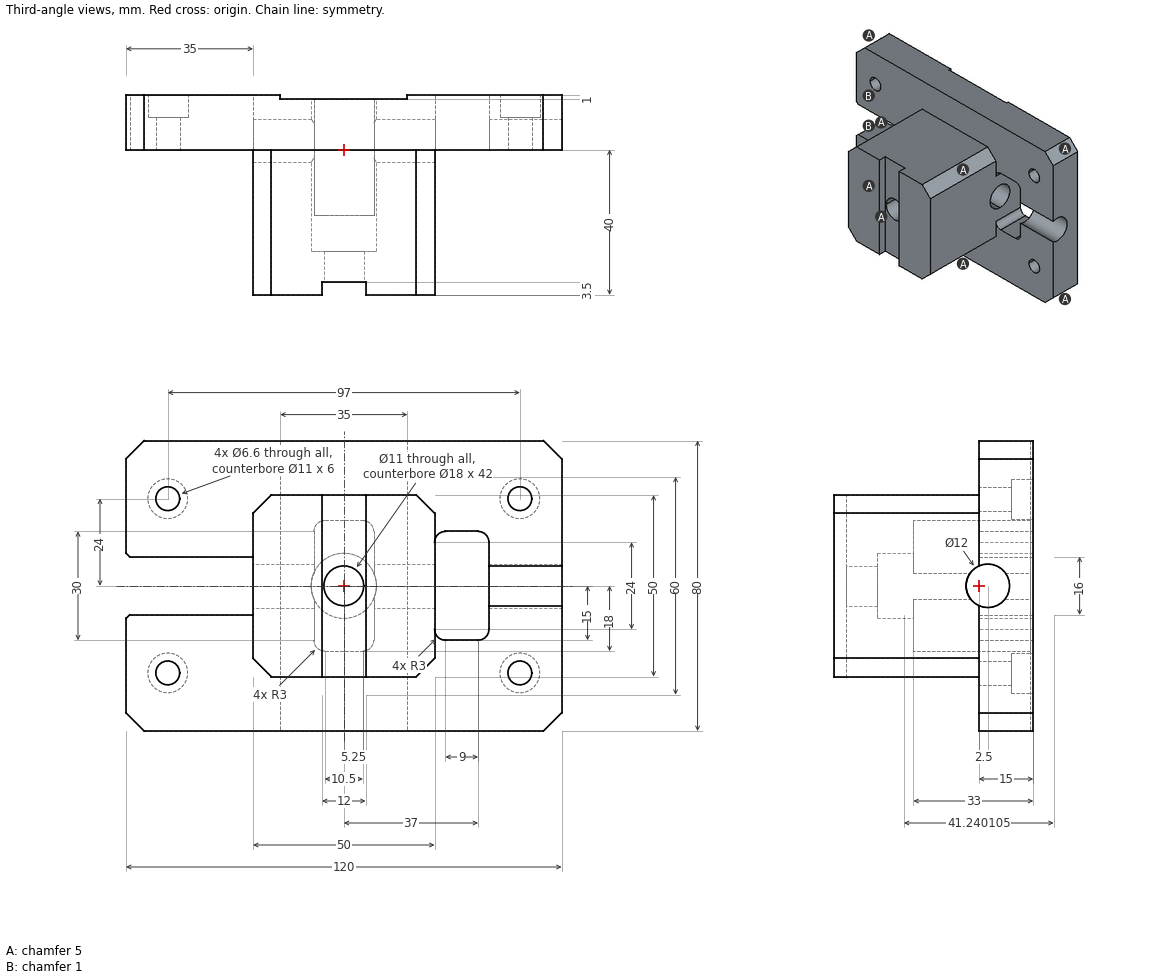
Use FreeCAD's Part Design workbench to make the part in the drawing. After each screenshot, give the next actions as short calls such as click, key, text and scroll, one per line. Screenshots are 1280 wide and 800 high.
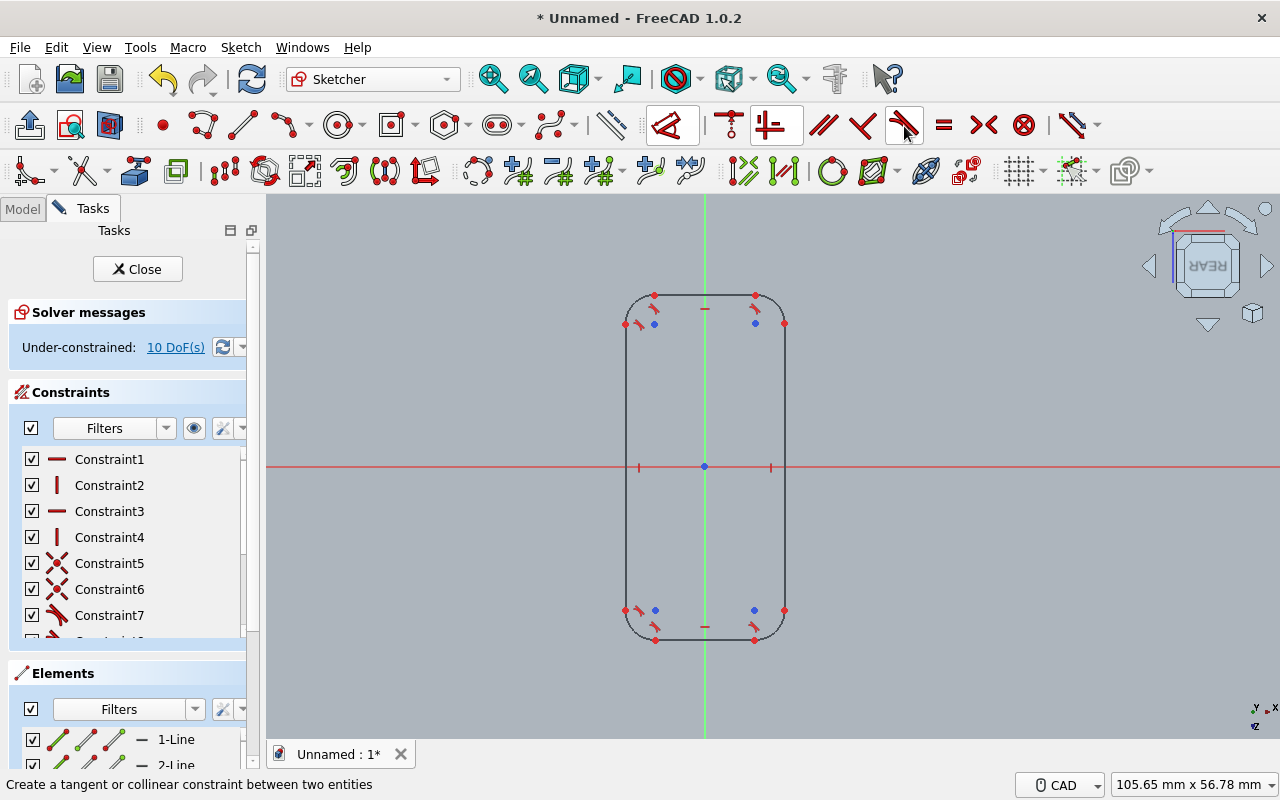
click(785, 525)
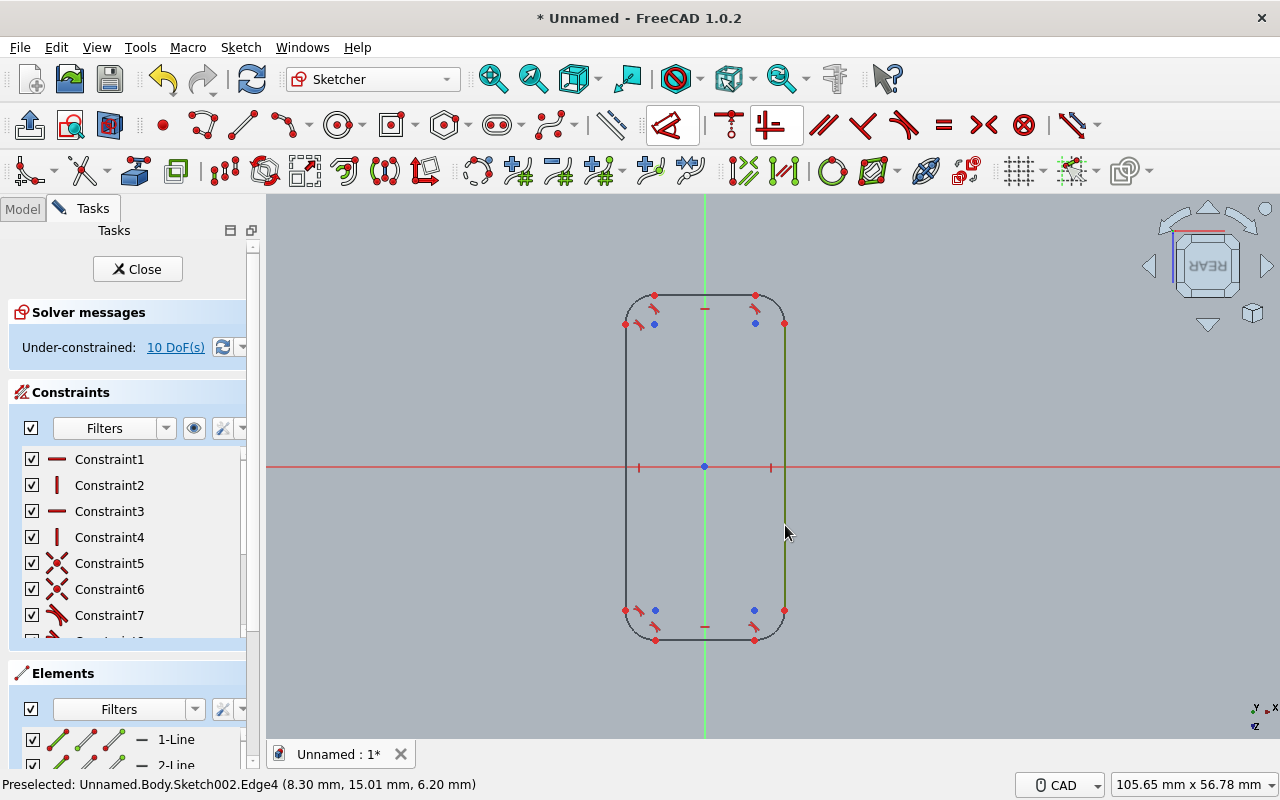
click(768, 637)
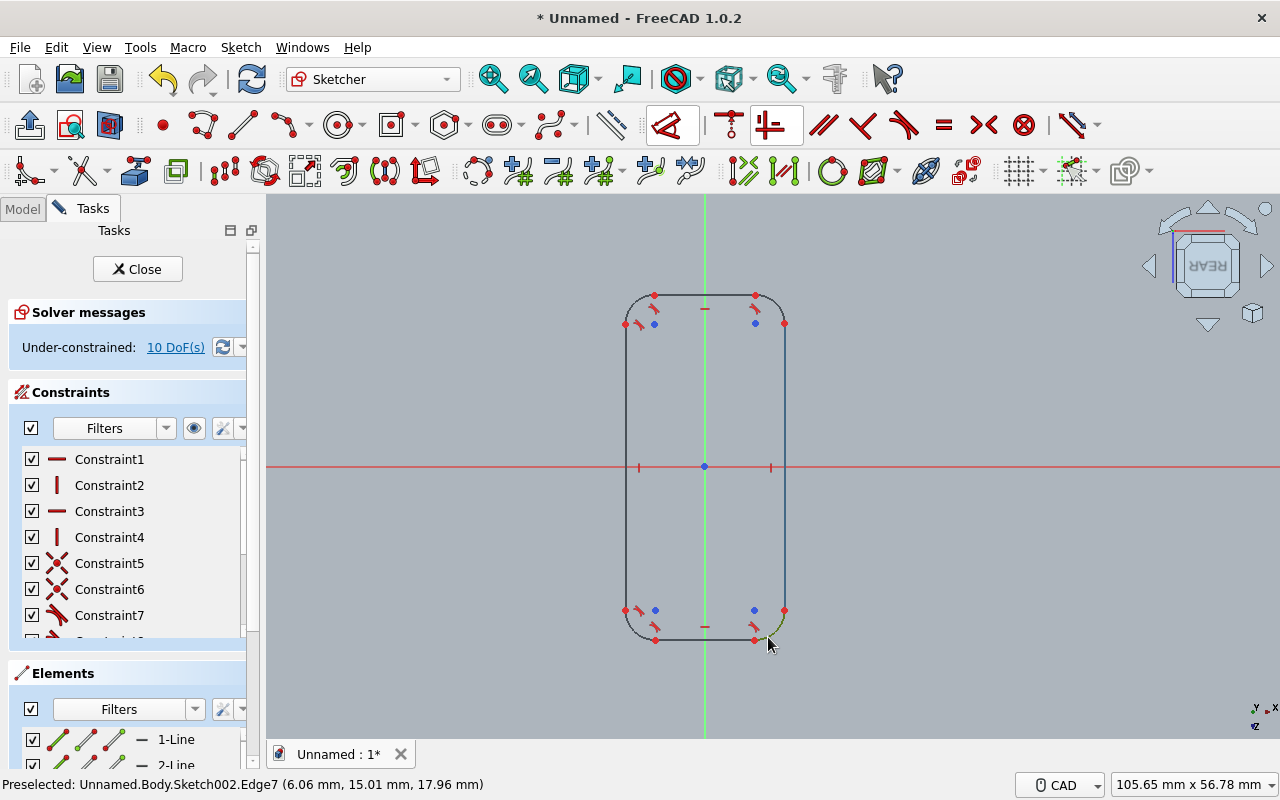
click(904, 126)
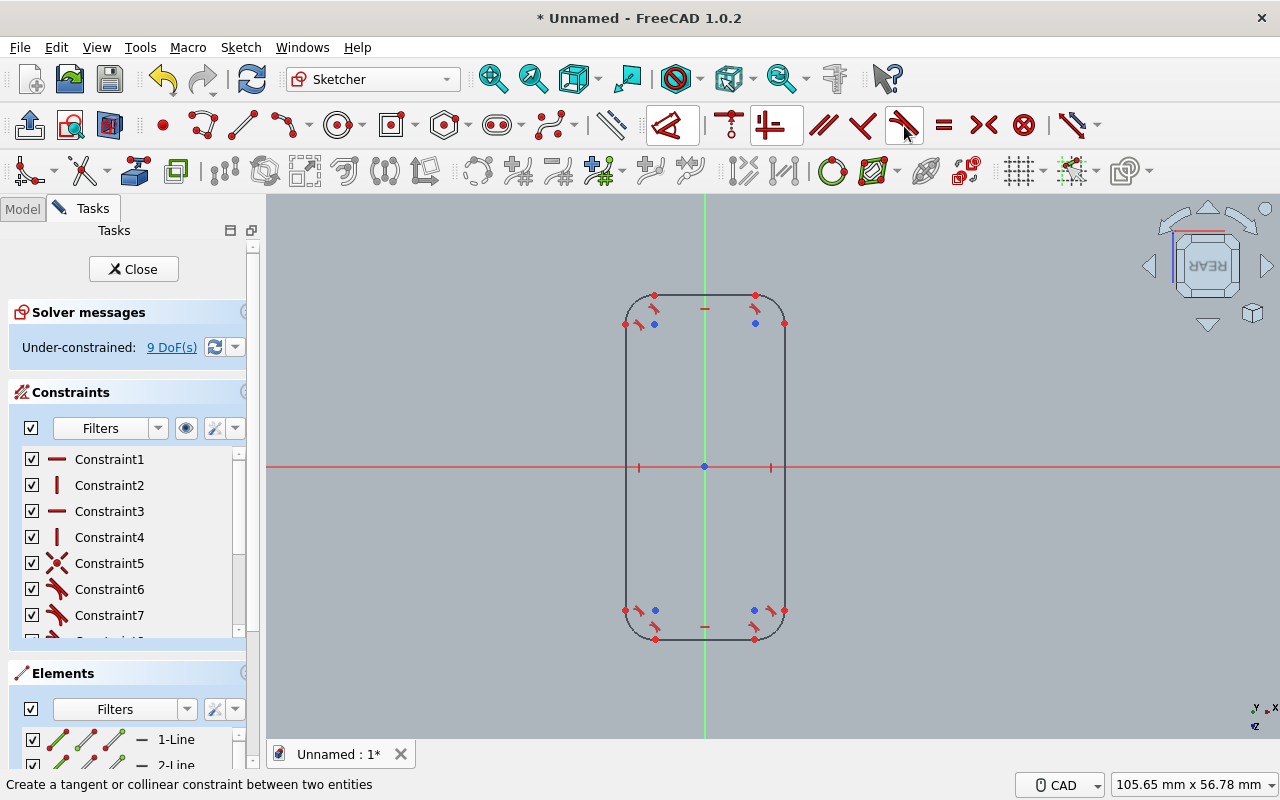
click(785, 524)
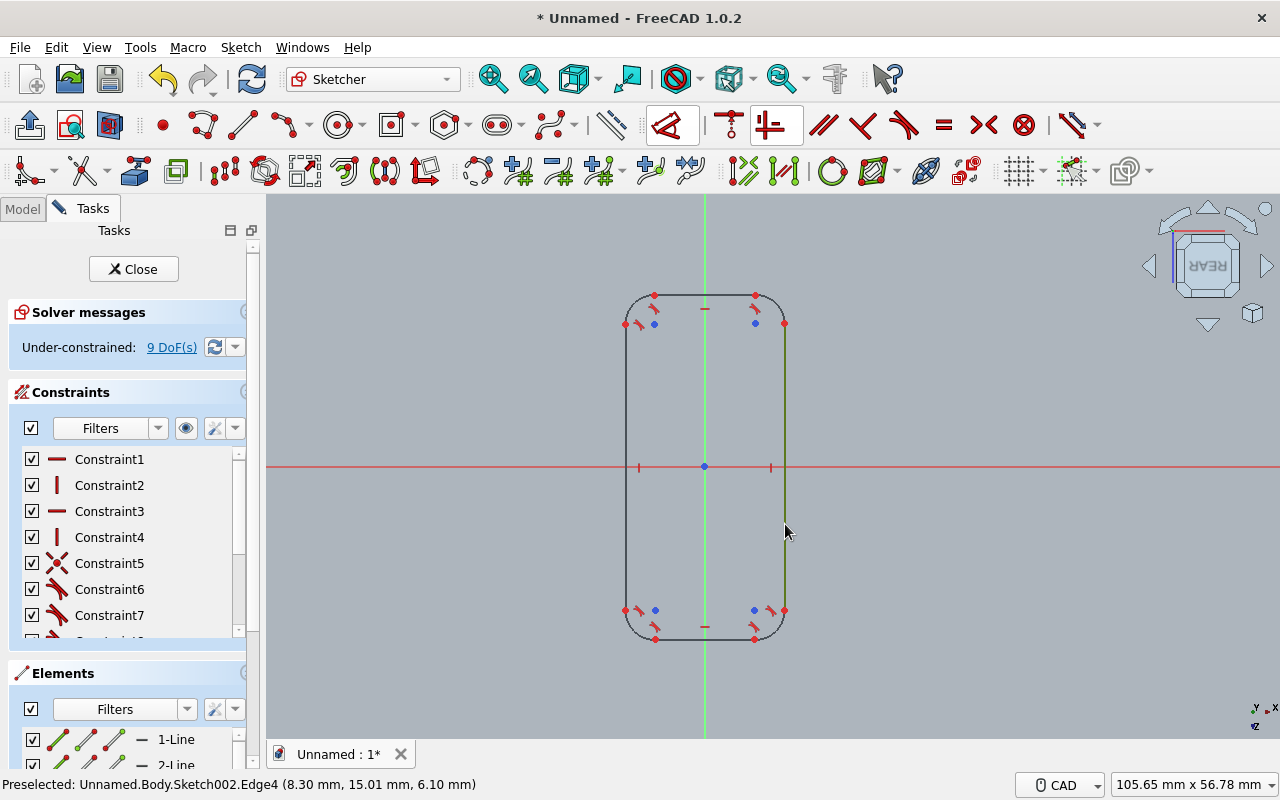
click(781, 311)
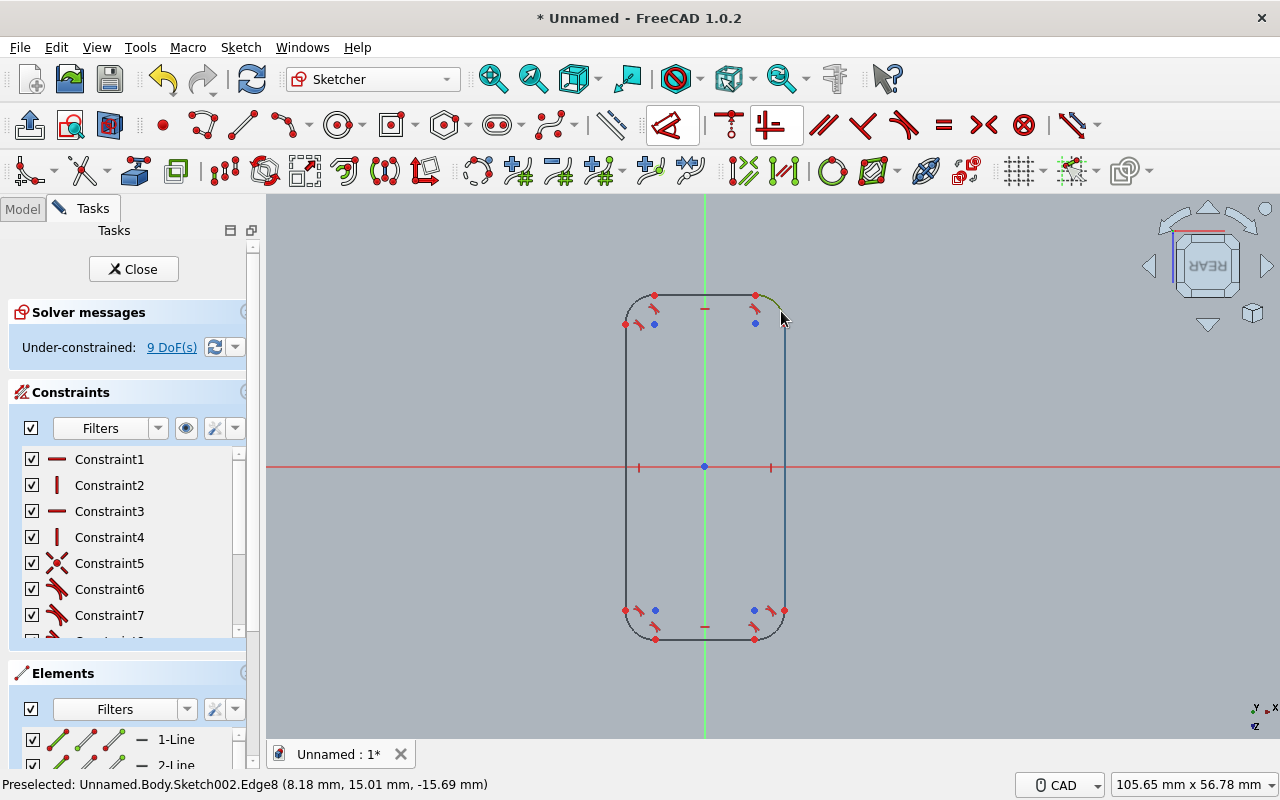
click(904, 126)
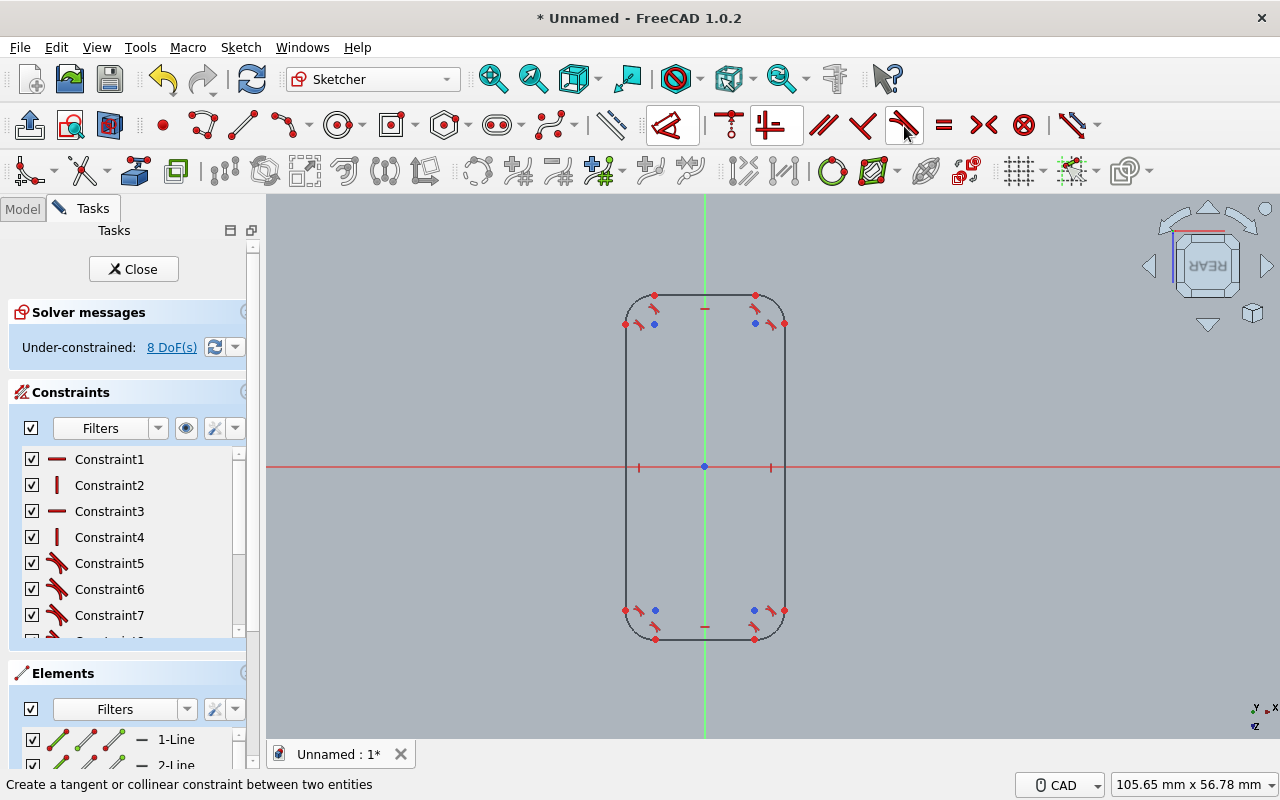
click(641, 298)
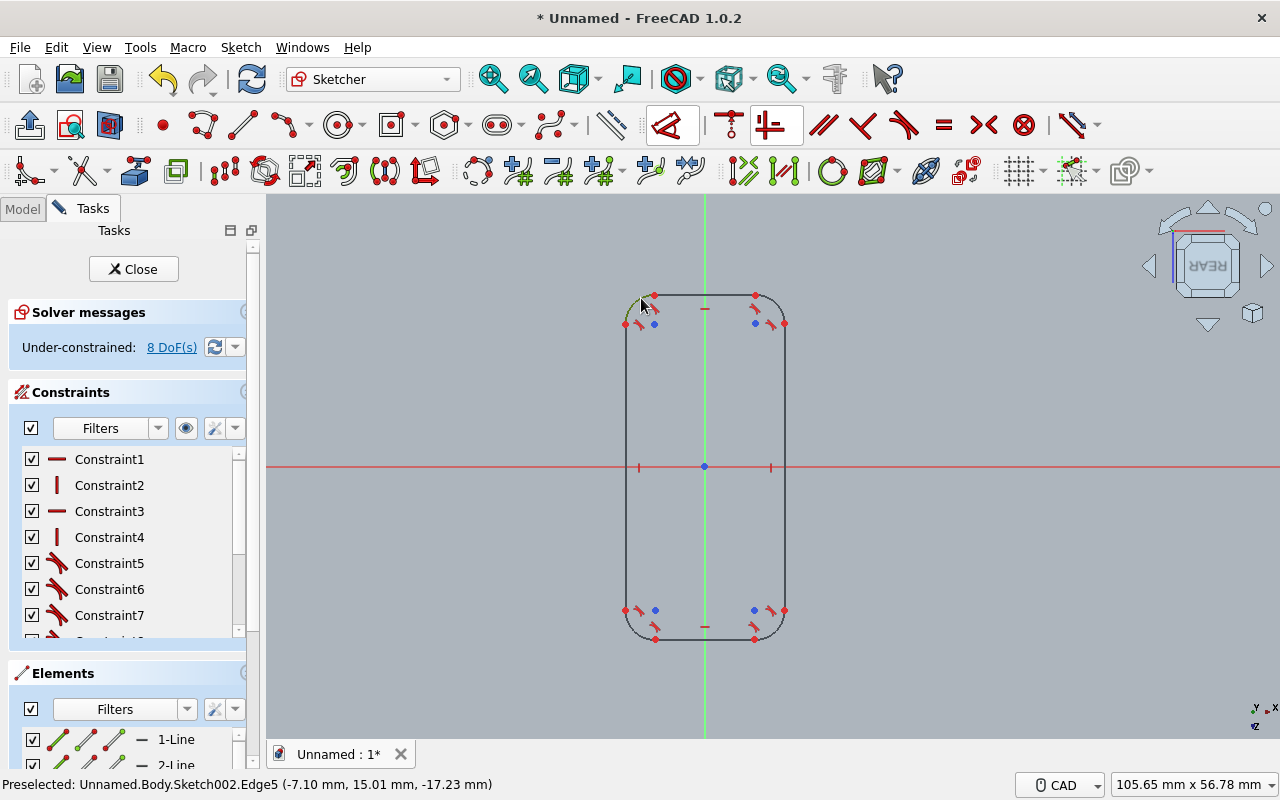
click(629, 624)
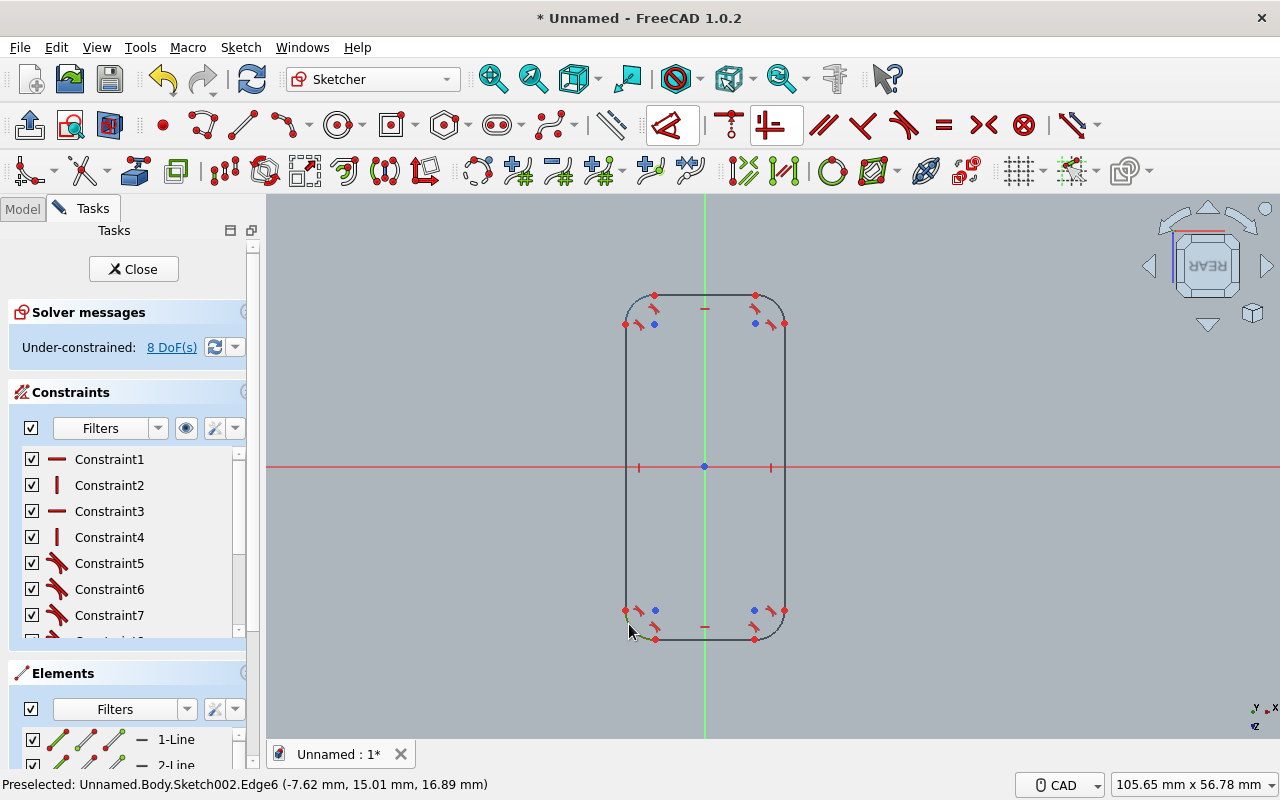
click(768, 637)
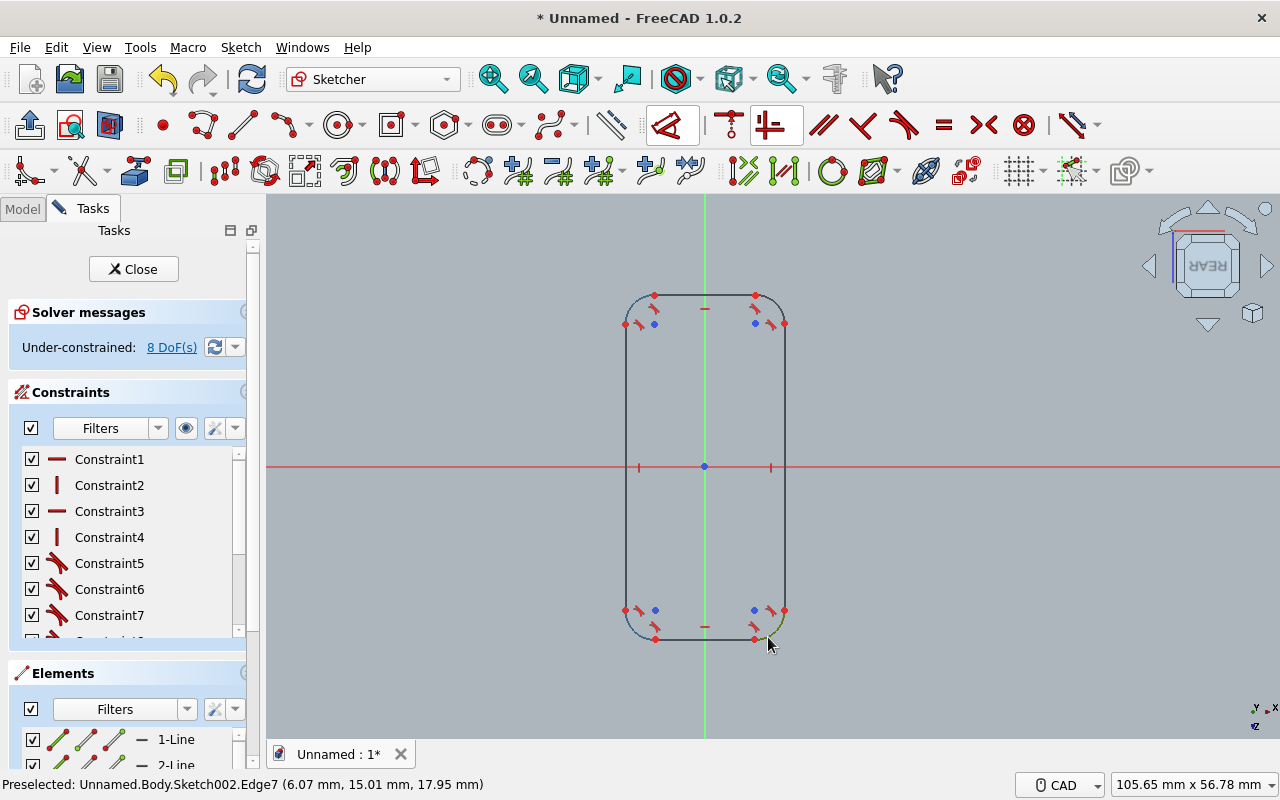
click(781, 311)